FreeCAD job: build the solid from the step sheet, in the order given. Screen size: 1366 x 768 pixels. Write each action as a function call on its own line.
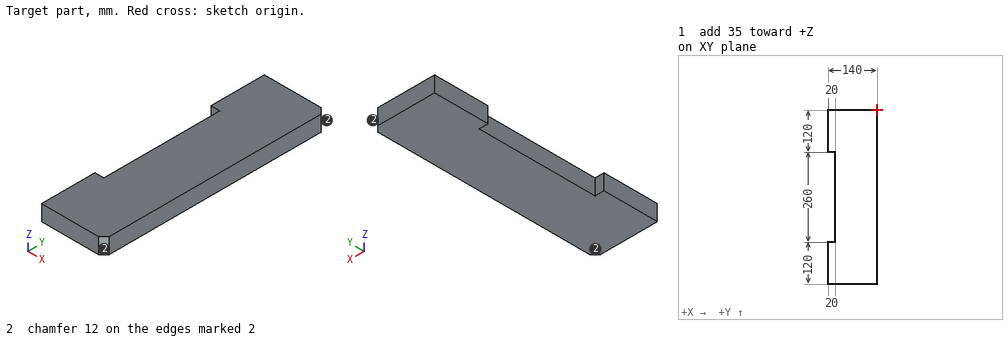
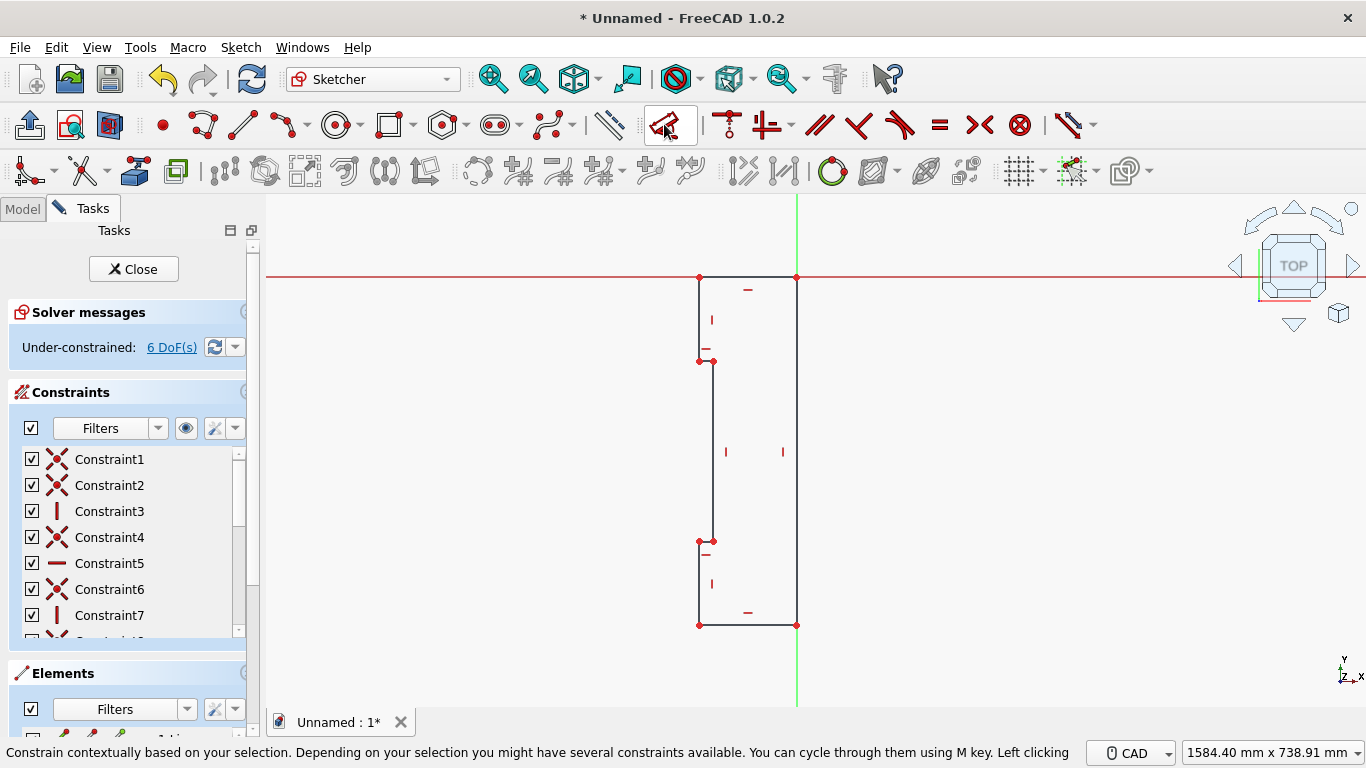
scroll(706, 361, up, 6)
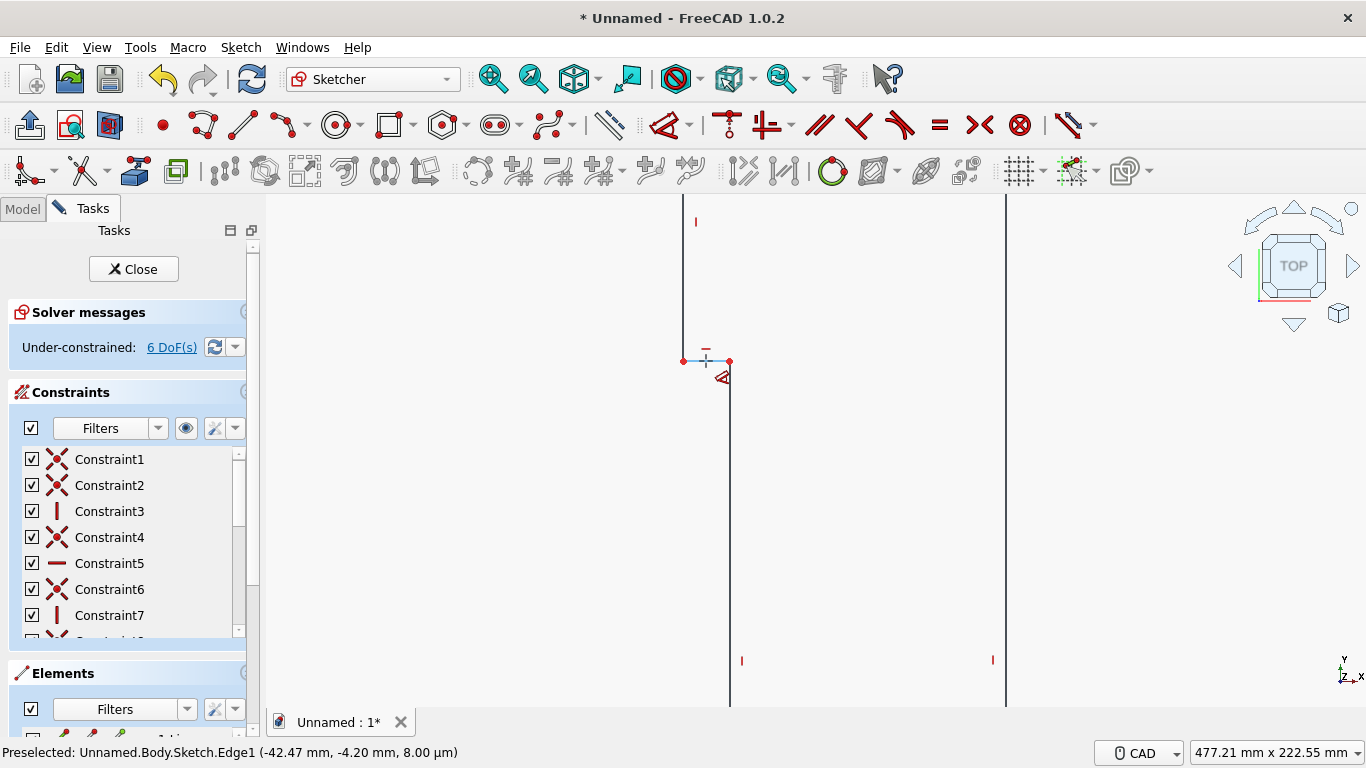
click(706, 361)
click(706, 327)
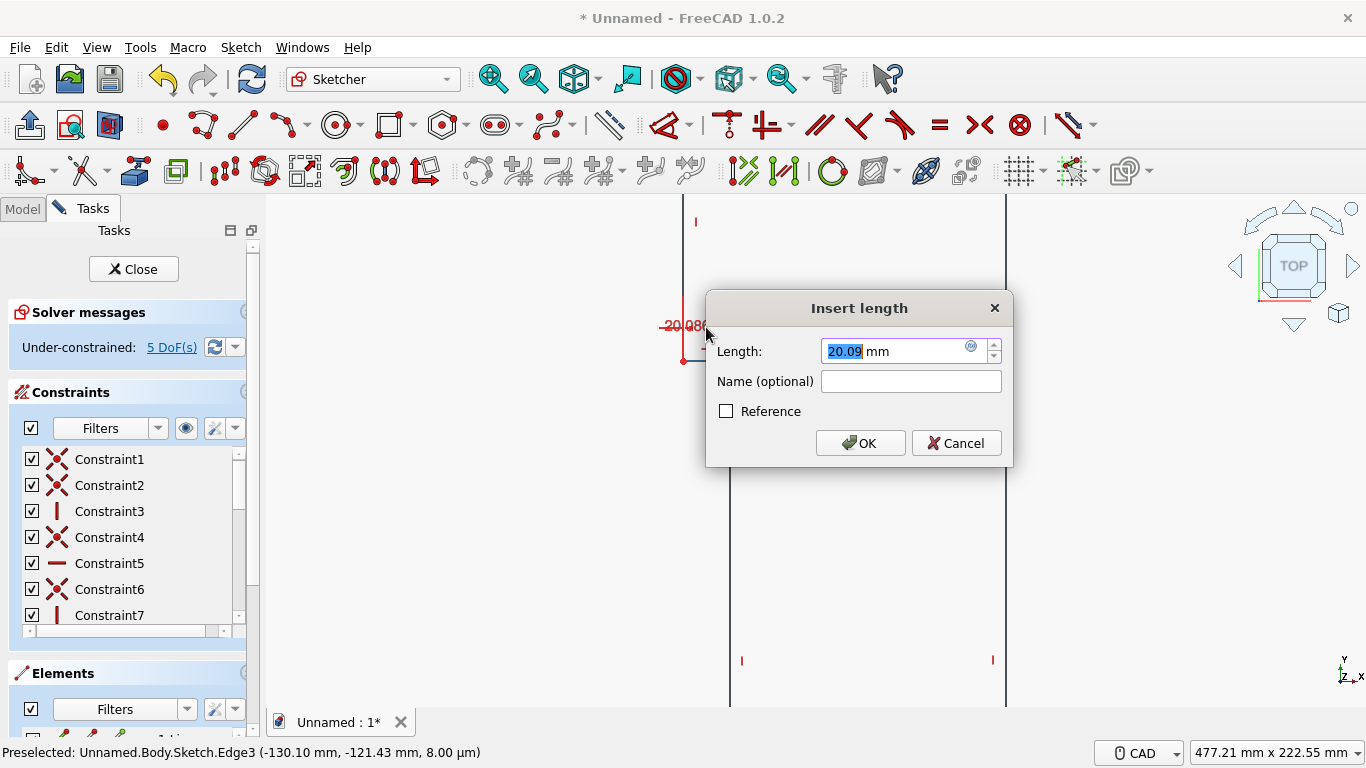
text(20)
key(Return)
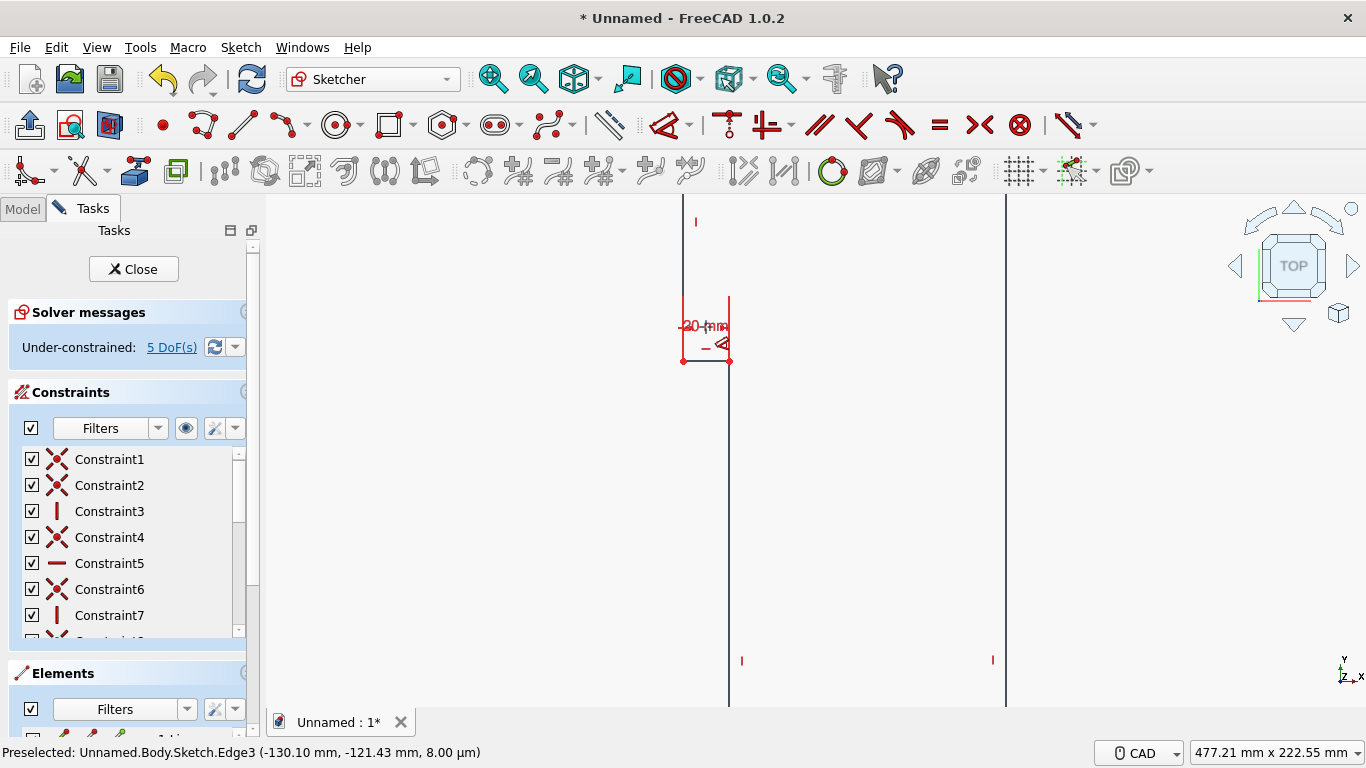
scroll(706, 361, down, 6)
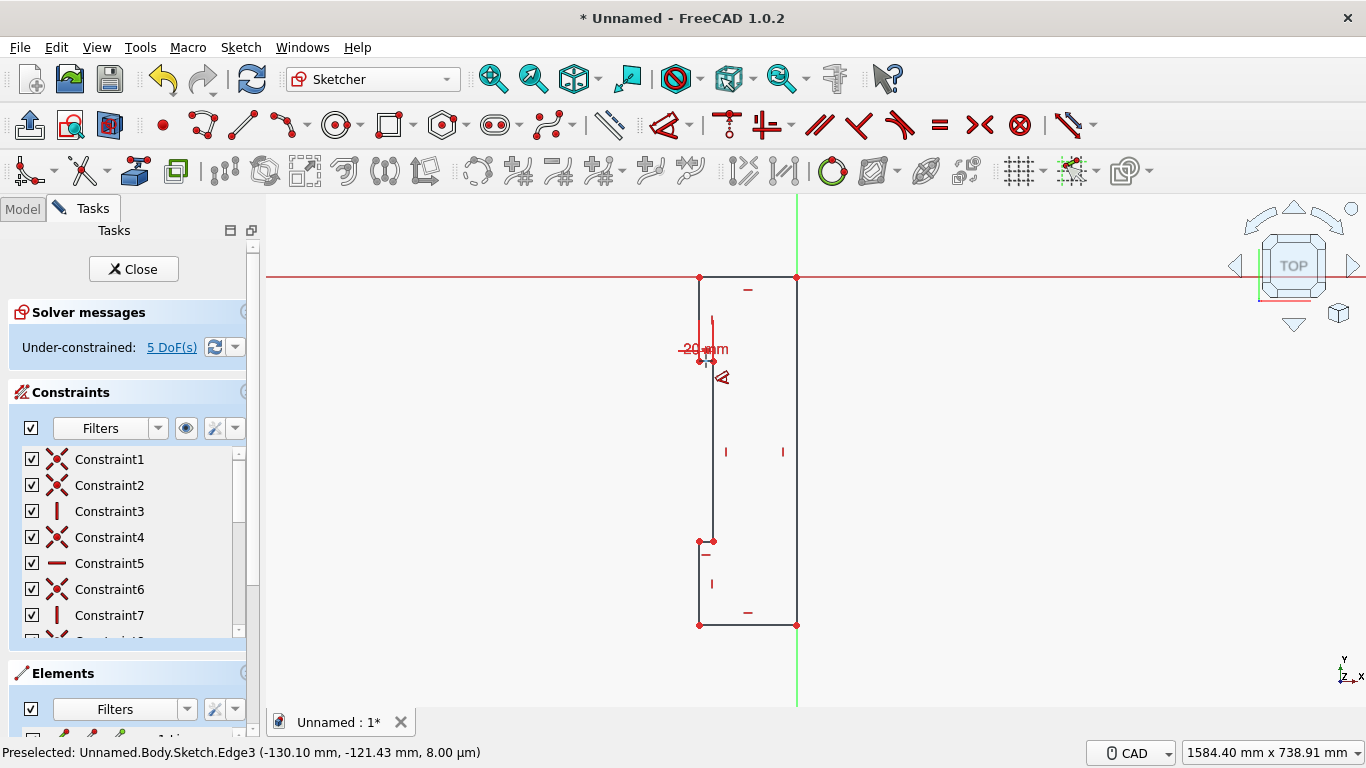
scroll(709, 542, up, 6)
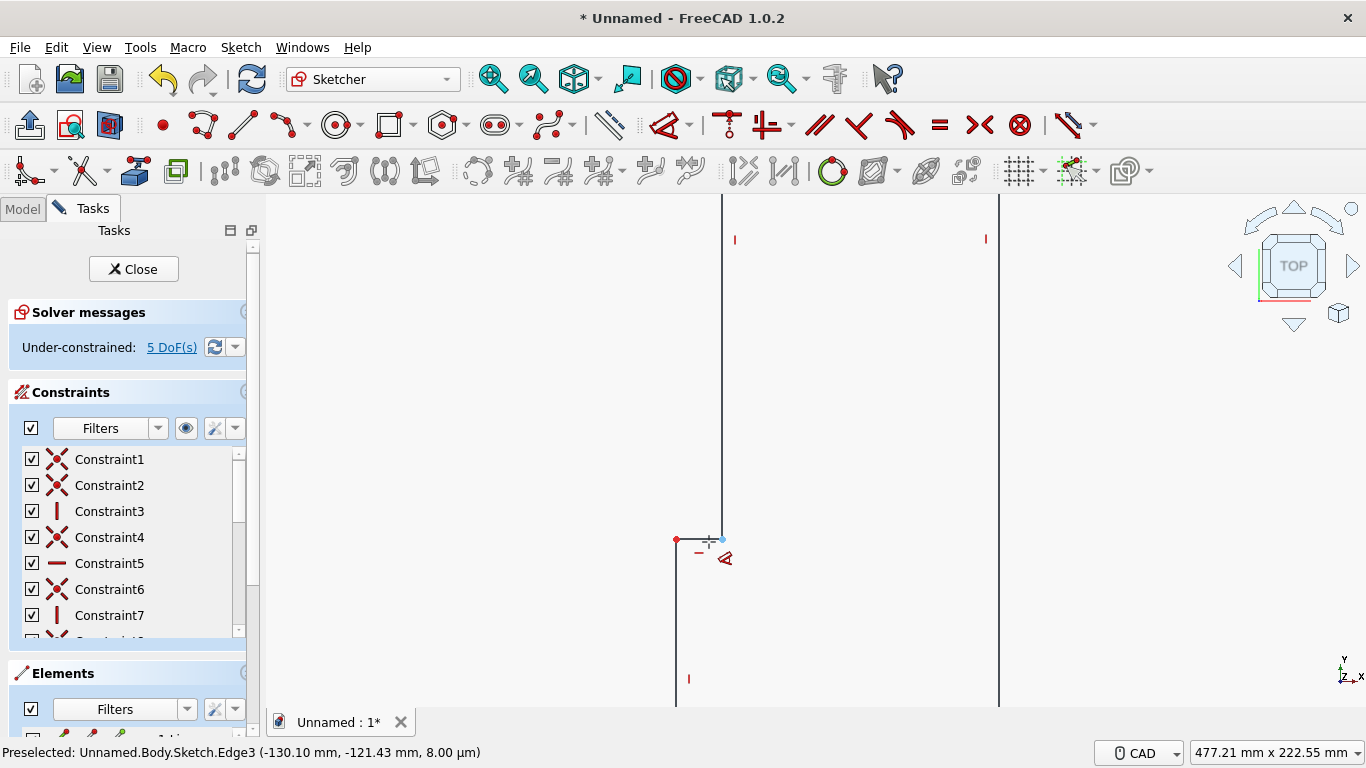
click(709, 539)
click(699, 573)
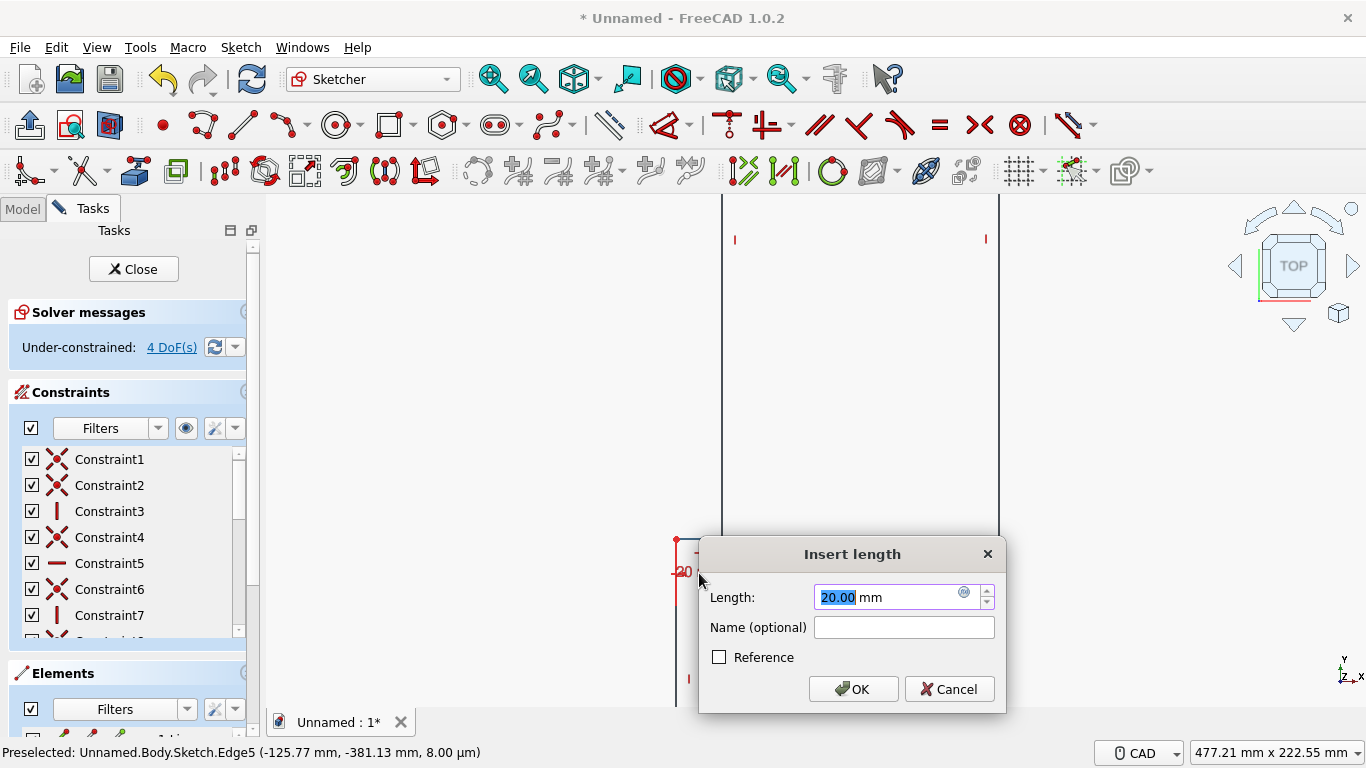
text(20)
key(Return)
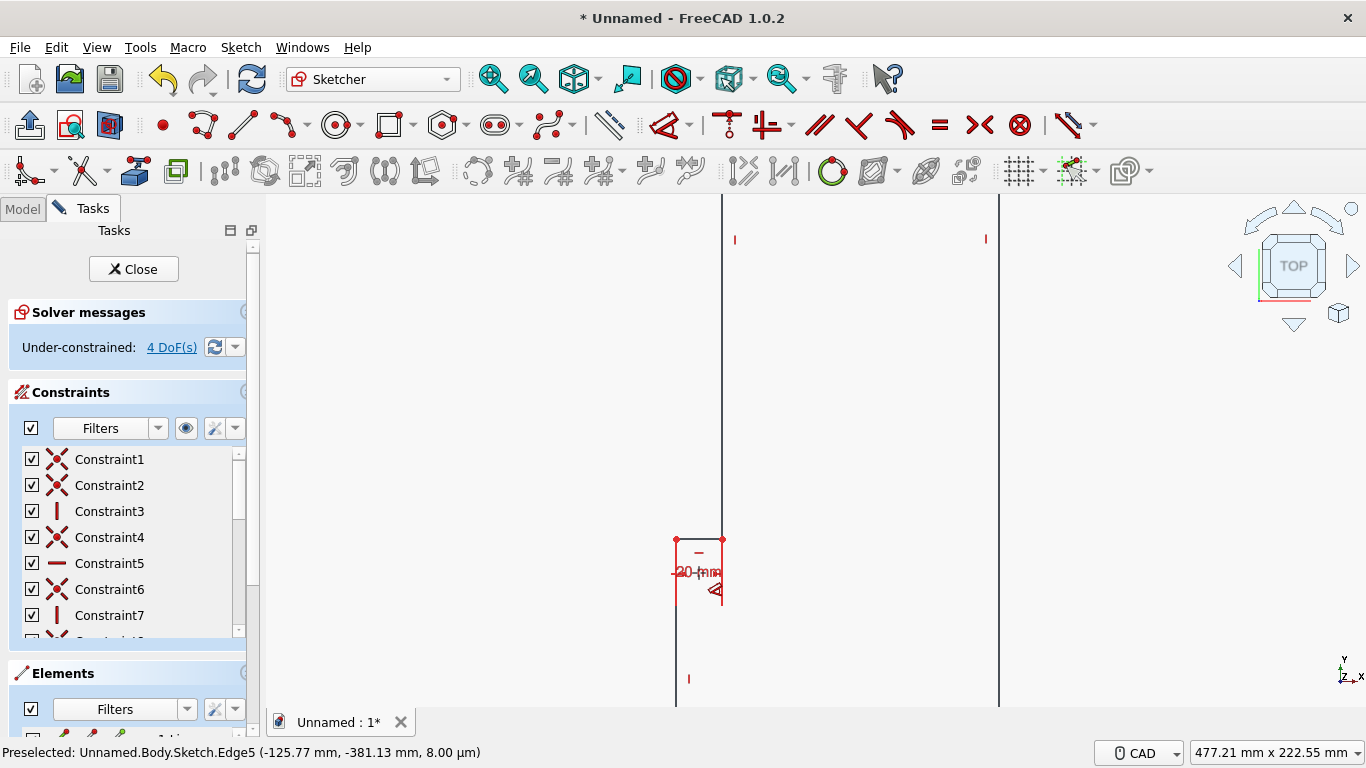
scroll(709, 543, down, 6)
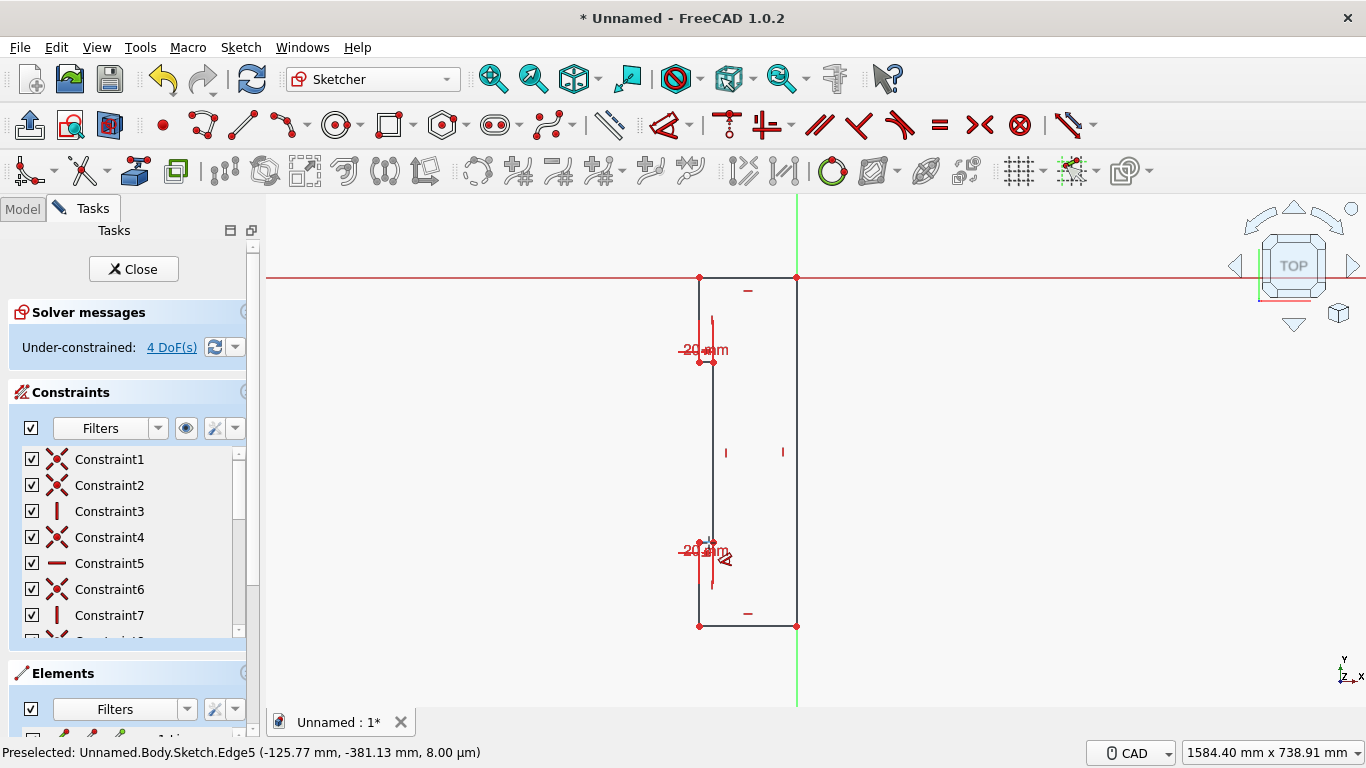
click(767, 278)
click(748, 244)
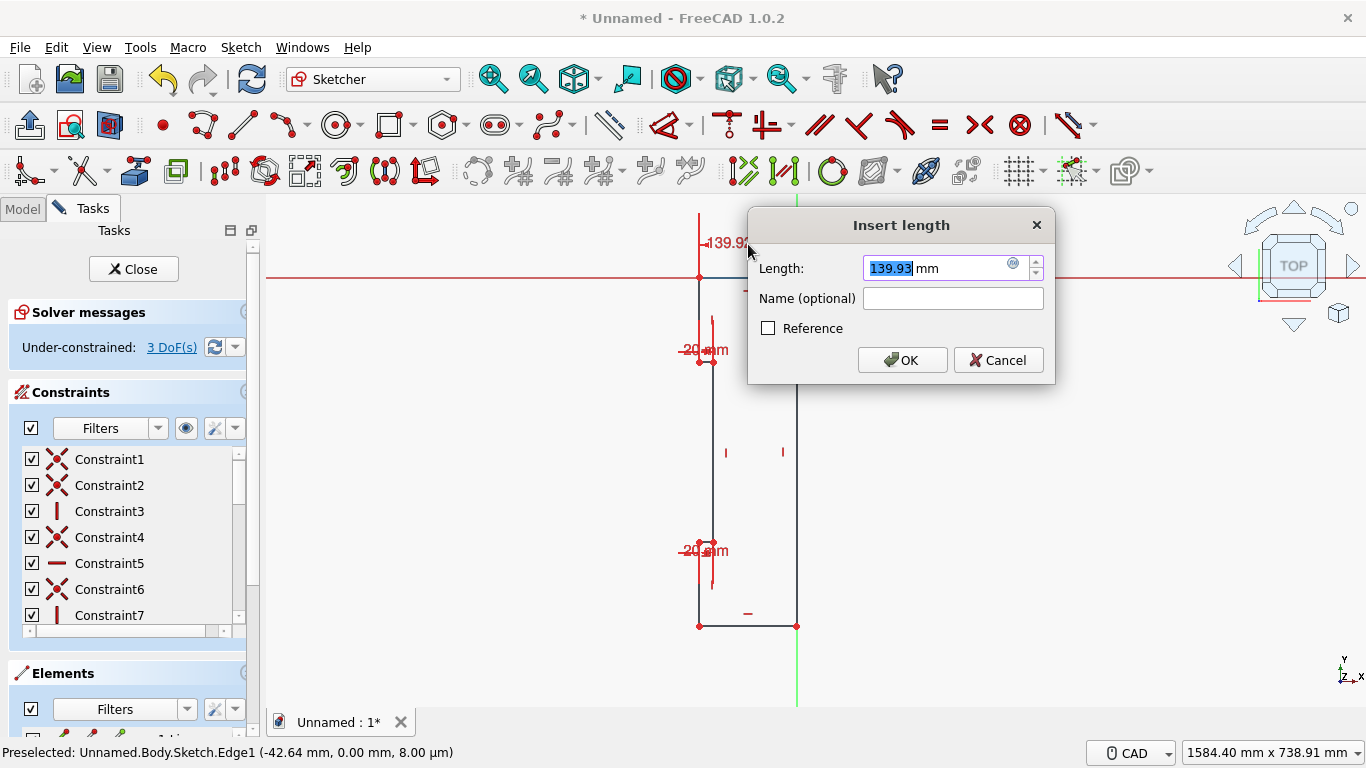
text(140)
key(Return)